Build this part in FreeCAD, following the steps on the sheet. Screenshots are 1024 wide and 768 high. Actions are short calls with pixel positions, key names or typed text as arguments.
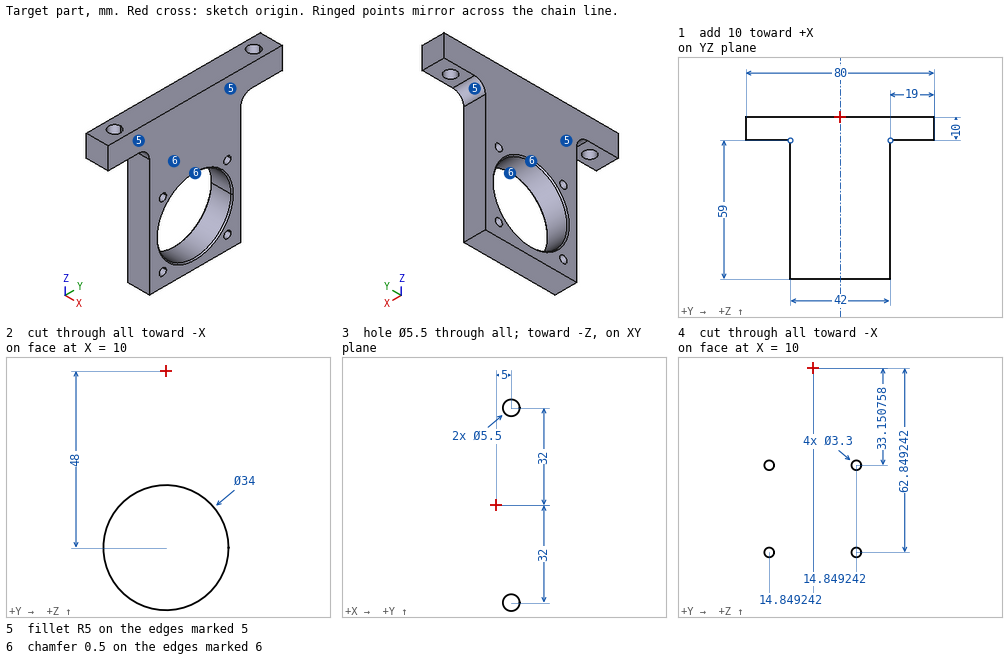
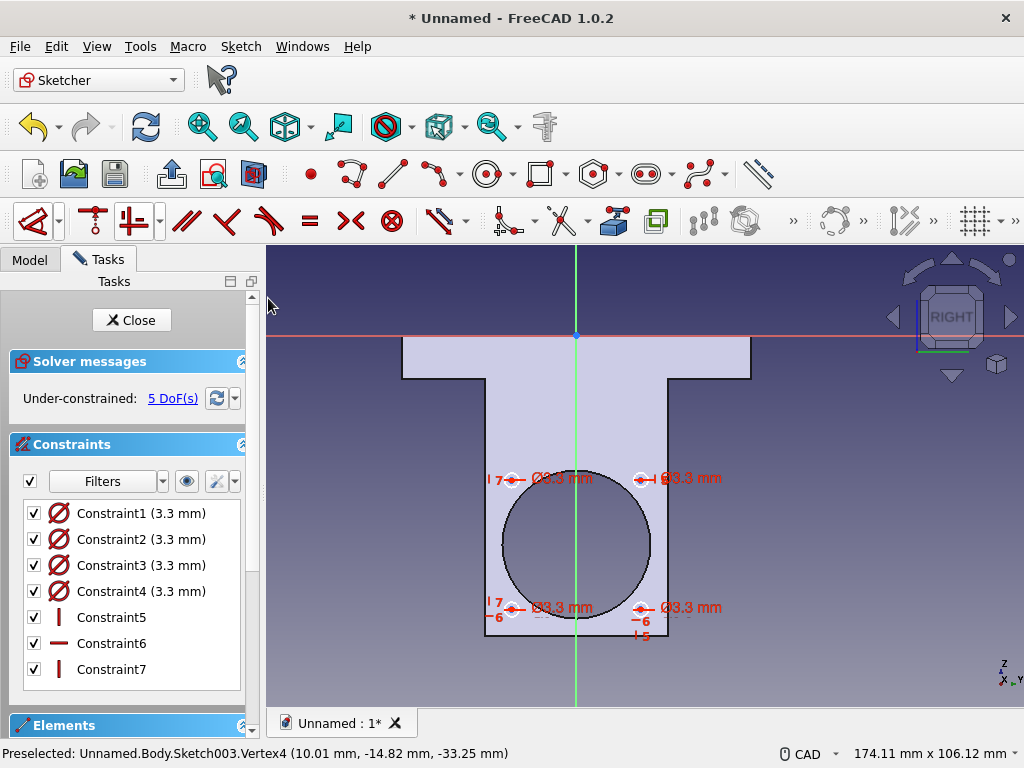
click(641, 480)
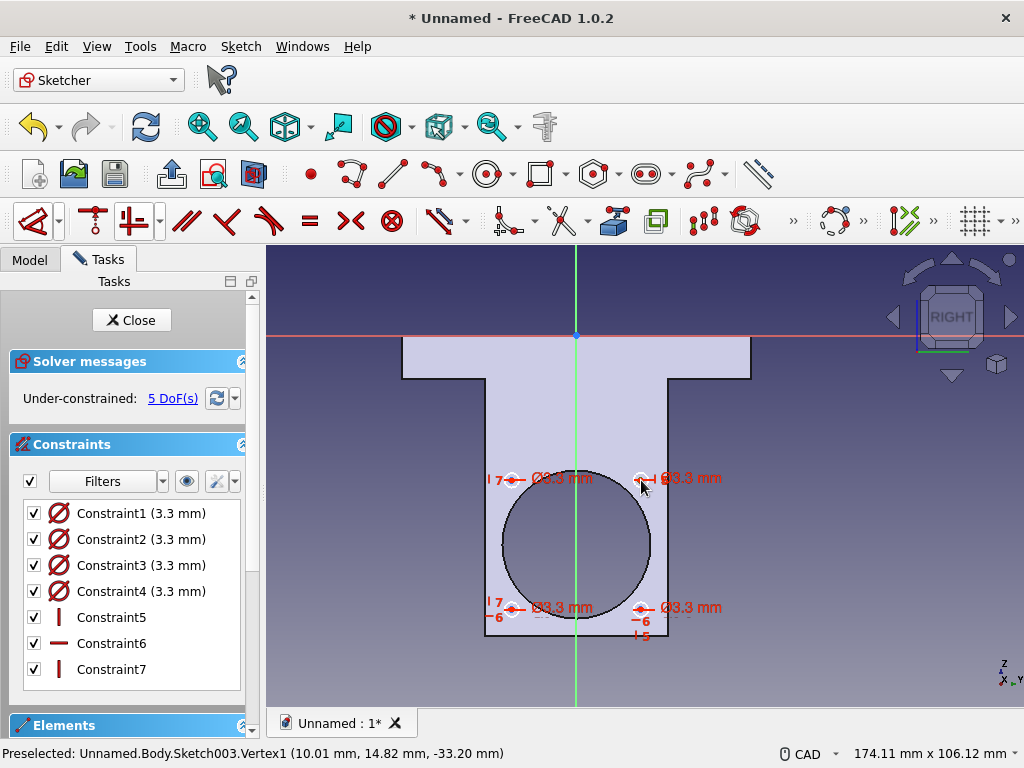
click(512, 480)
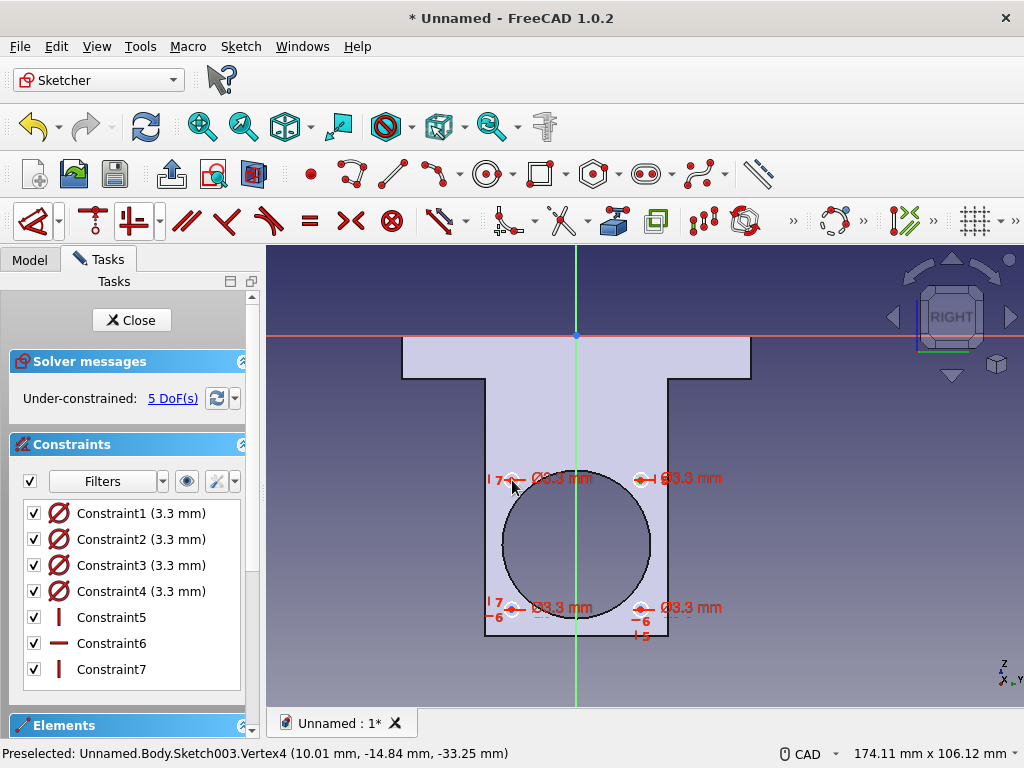
click(160, 222)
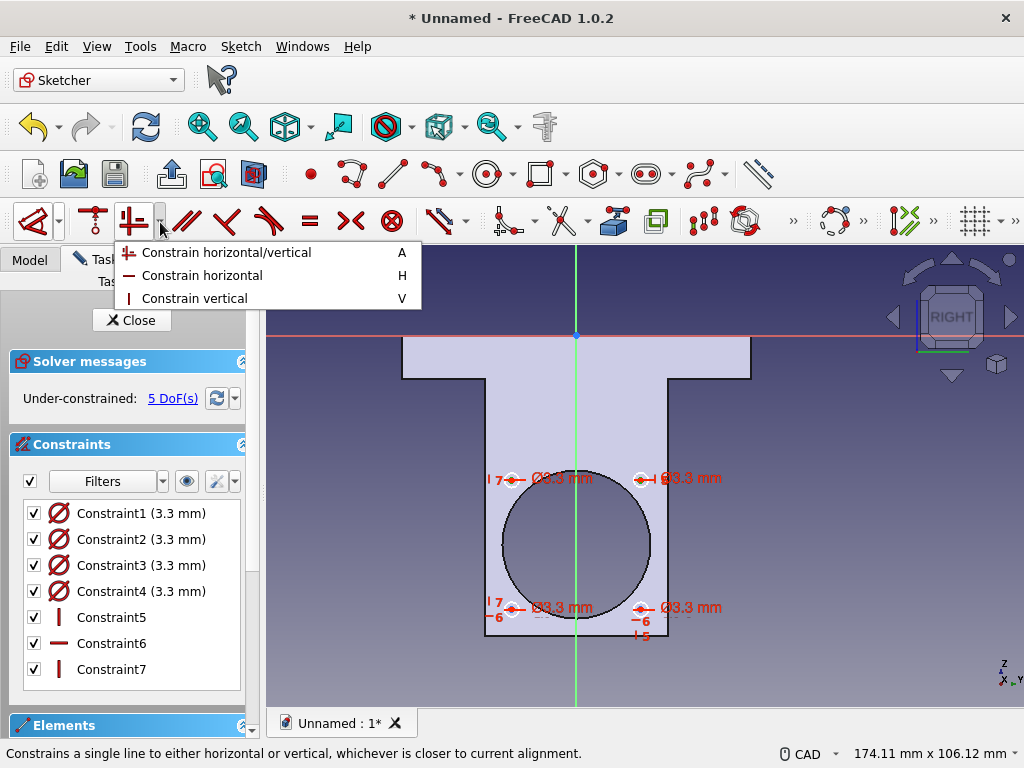
click(268, 276)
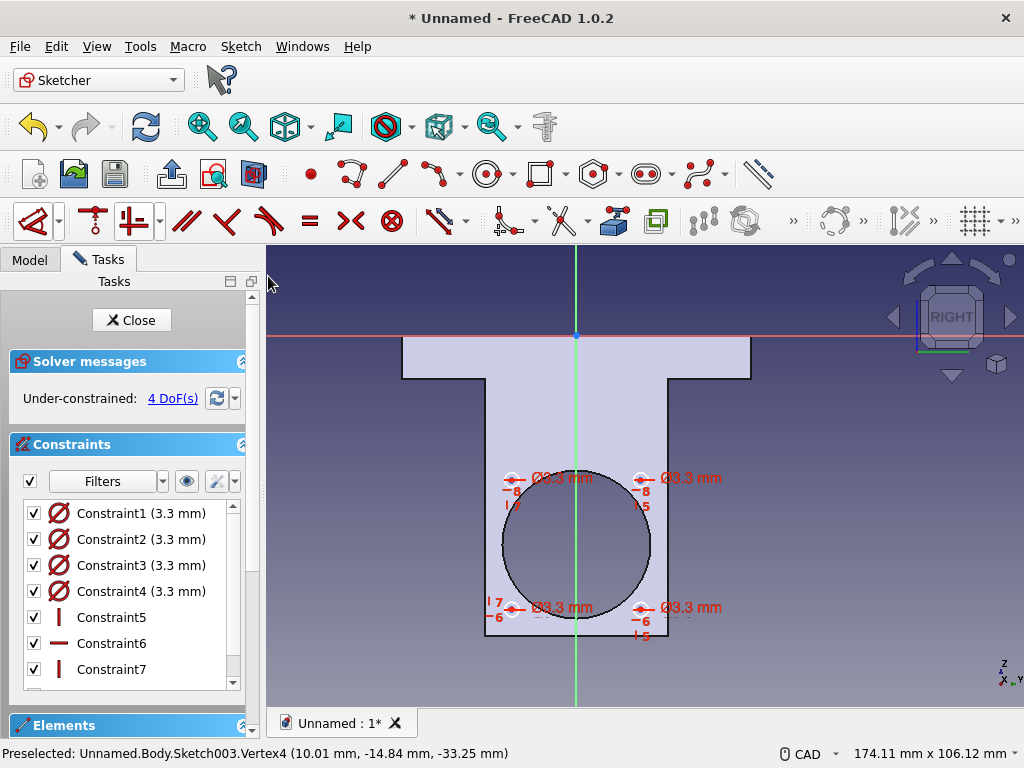
click(641, 480)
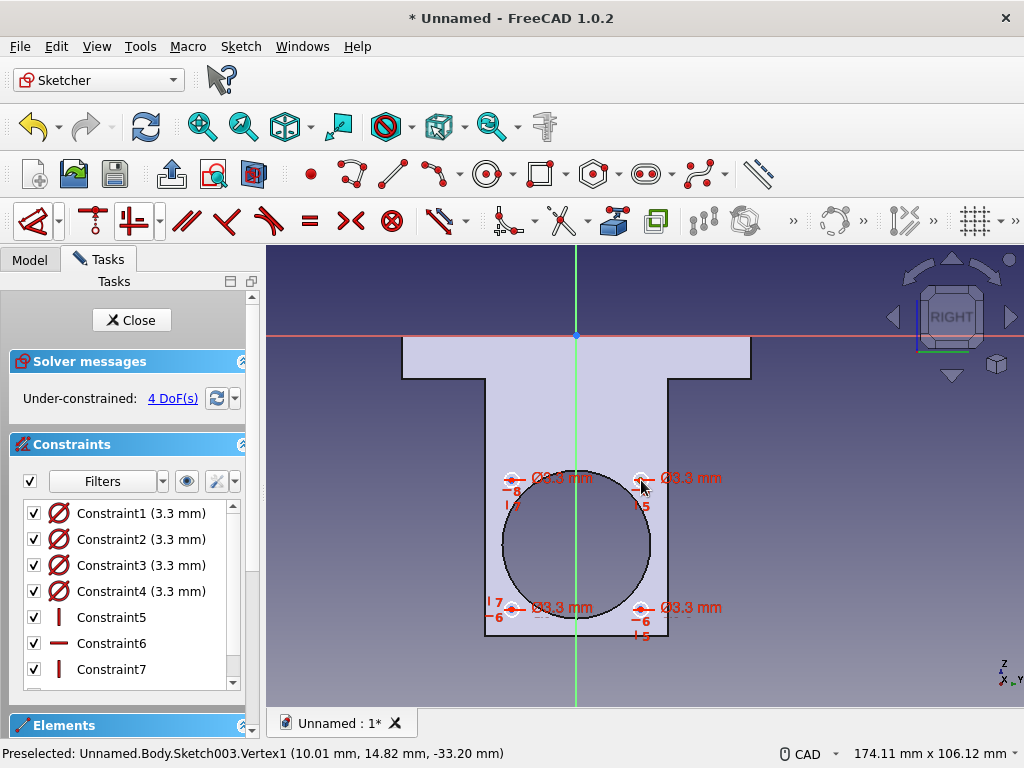
click(58, 222)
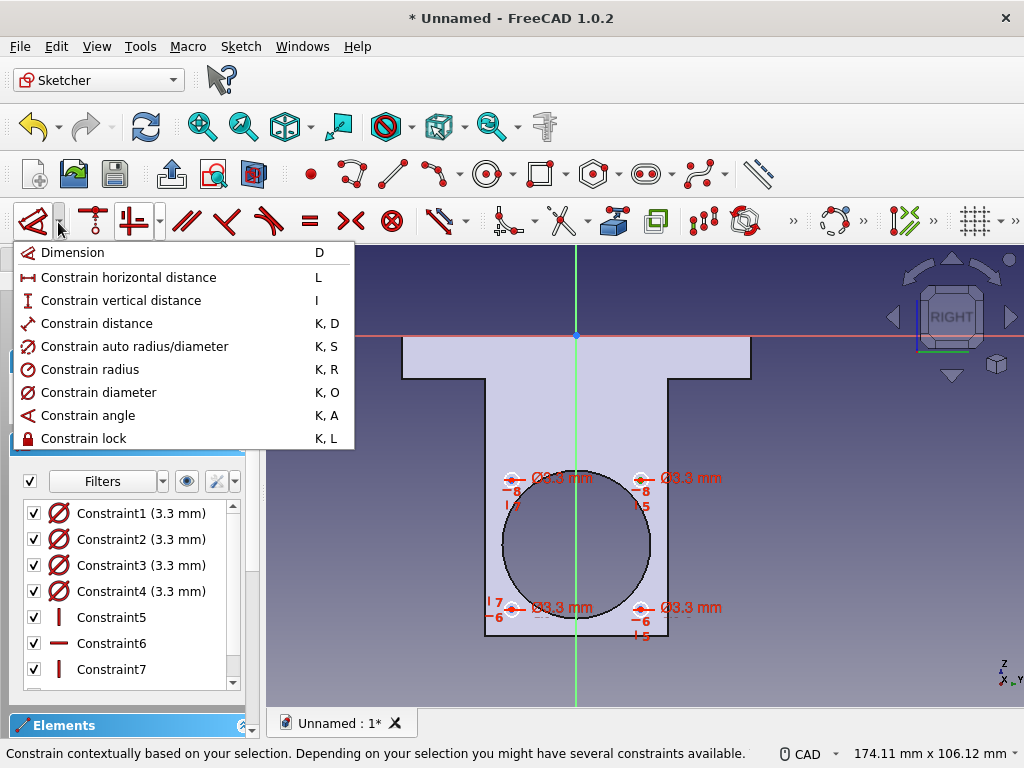
click(184, 278)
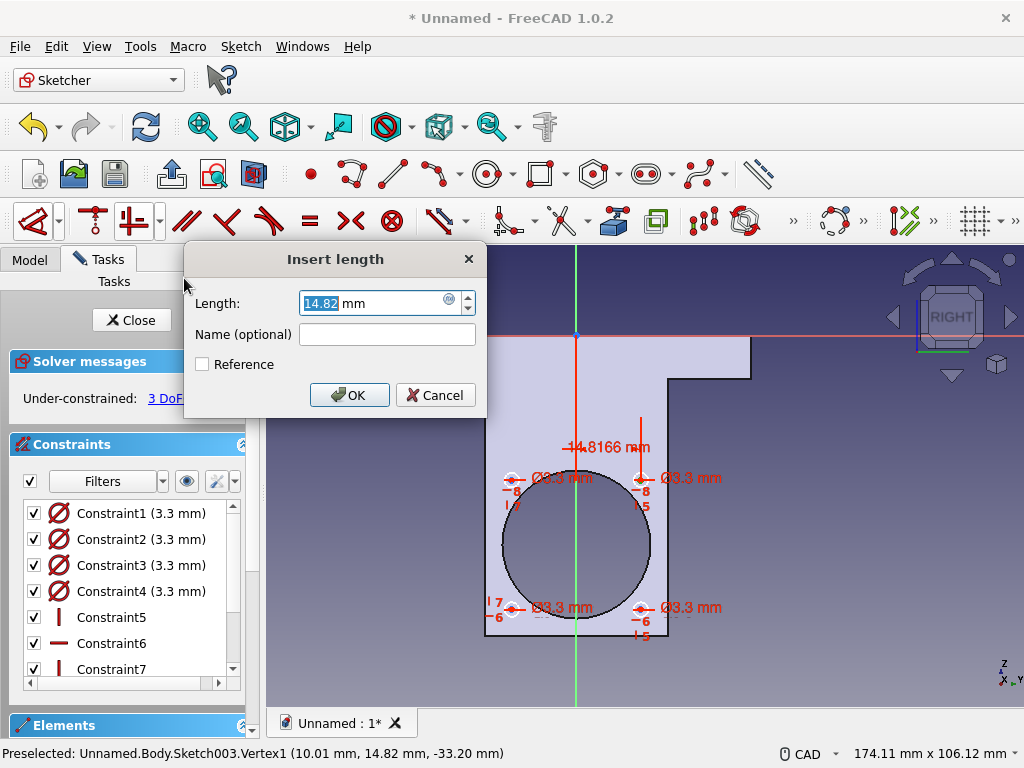
text(14.849242)
key(Return)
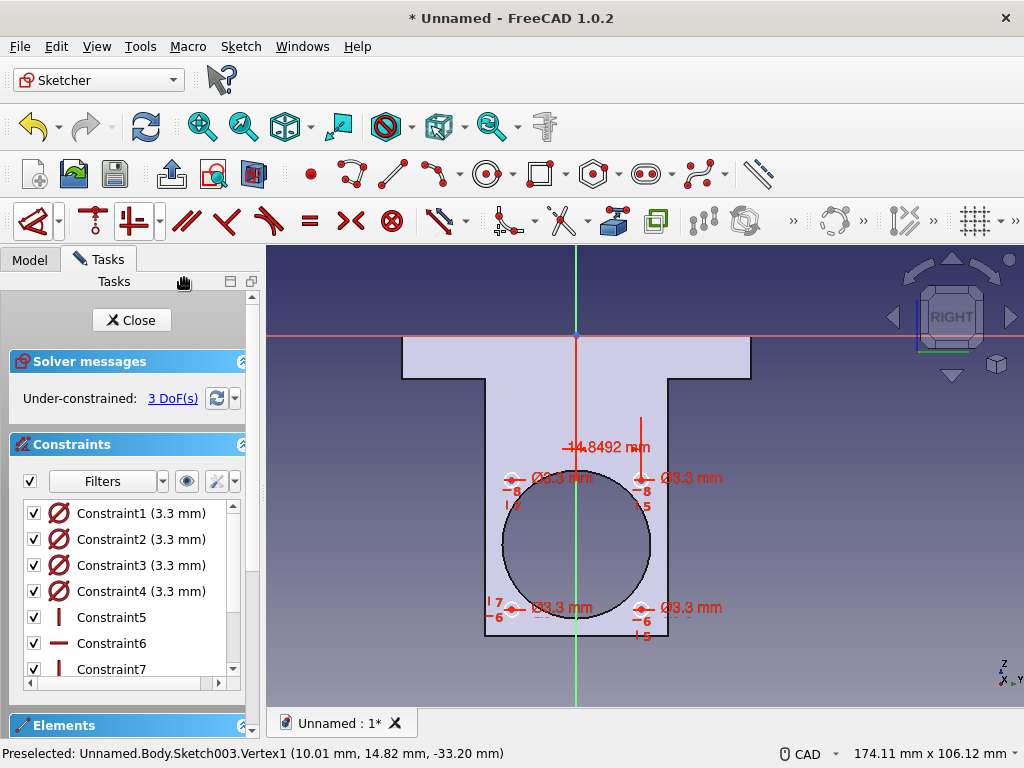
click(641, 480)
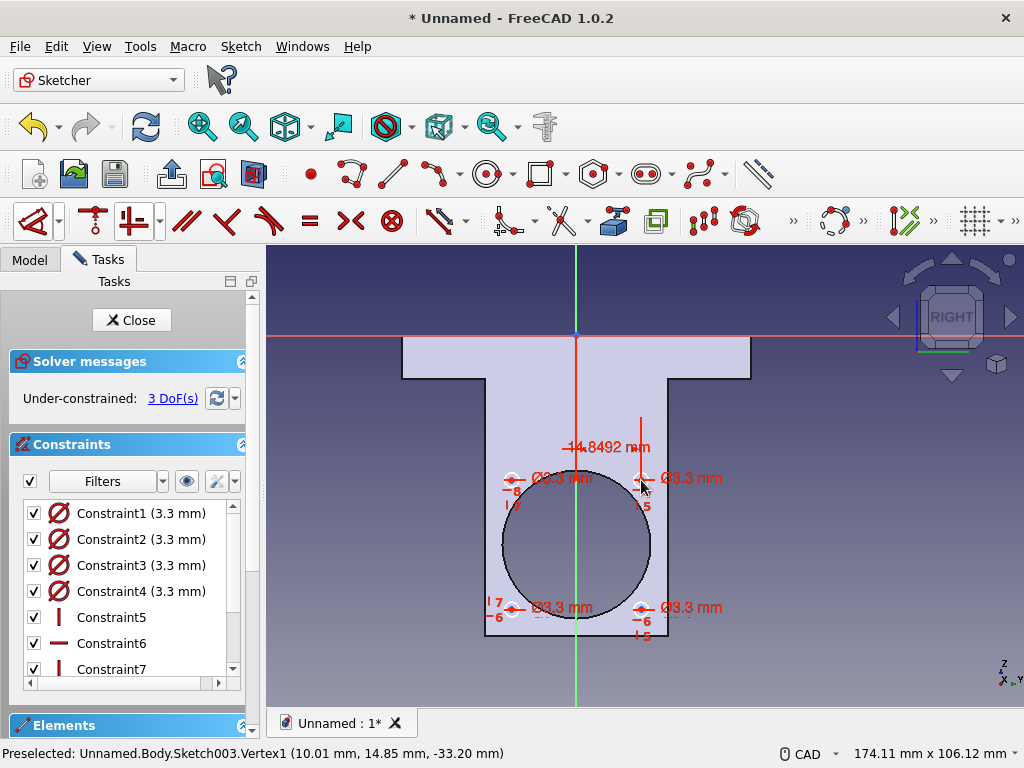
key(i)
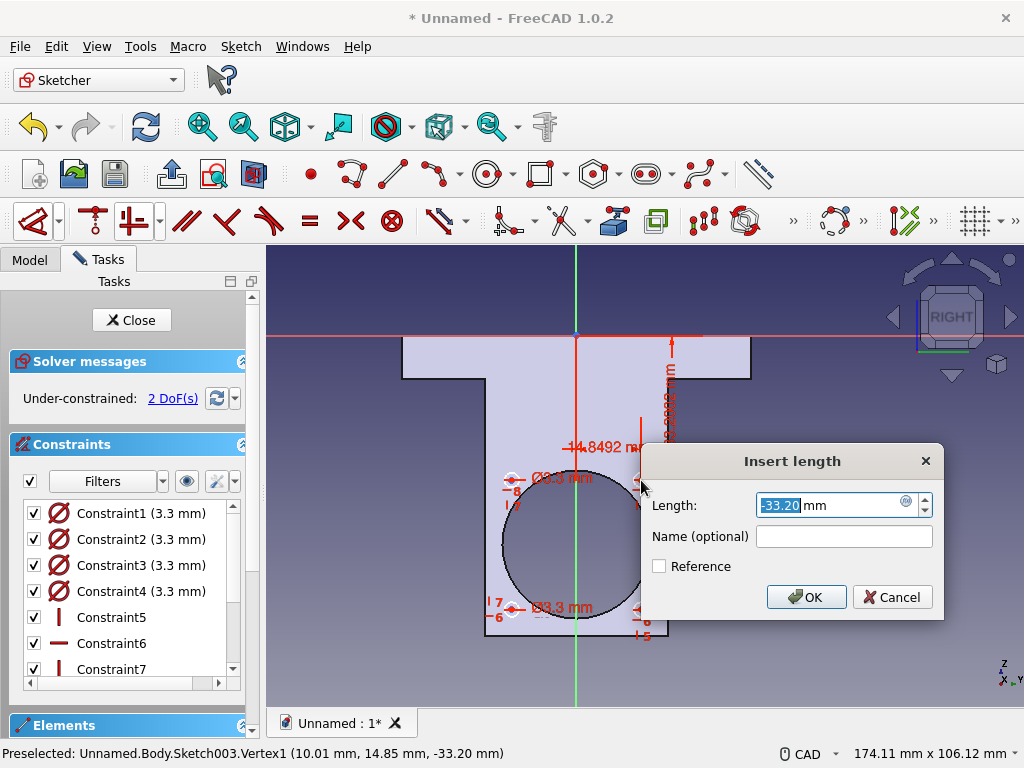
text(-33.150758)
key(Return)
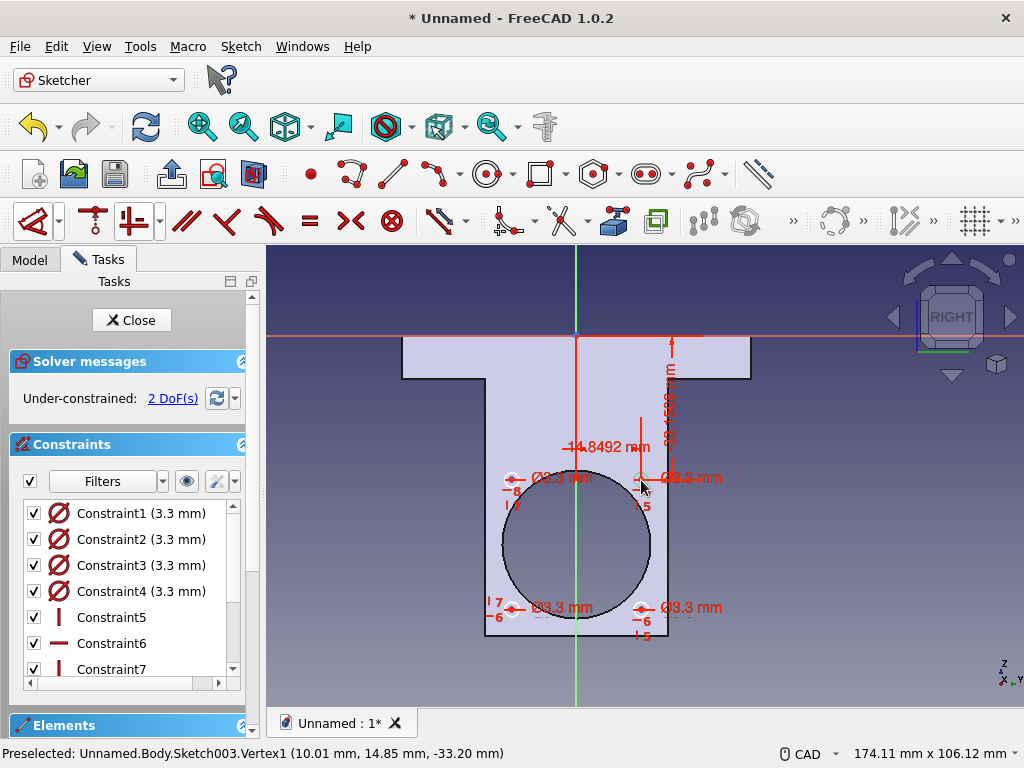
click(641, 610)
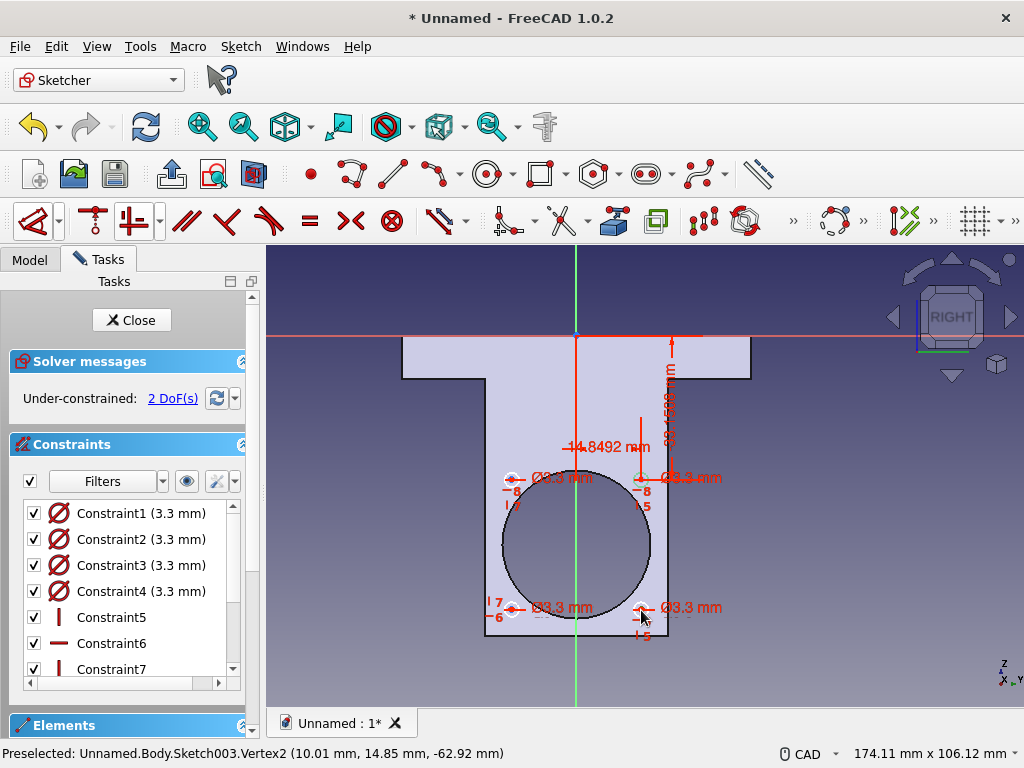
key(i)